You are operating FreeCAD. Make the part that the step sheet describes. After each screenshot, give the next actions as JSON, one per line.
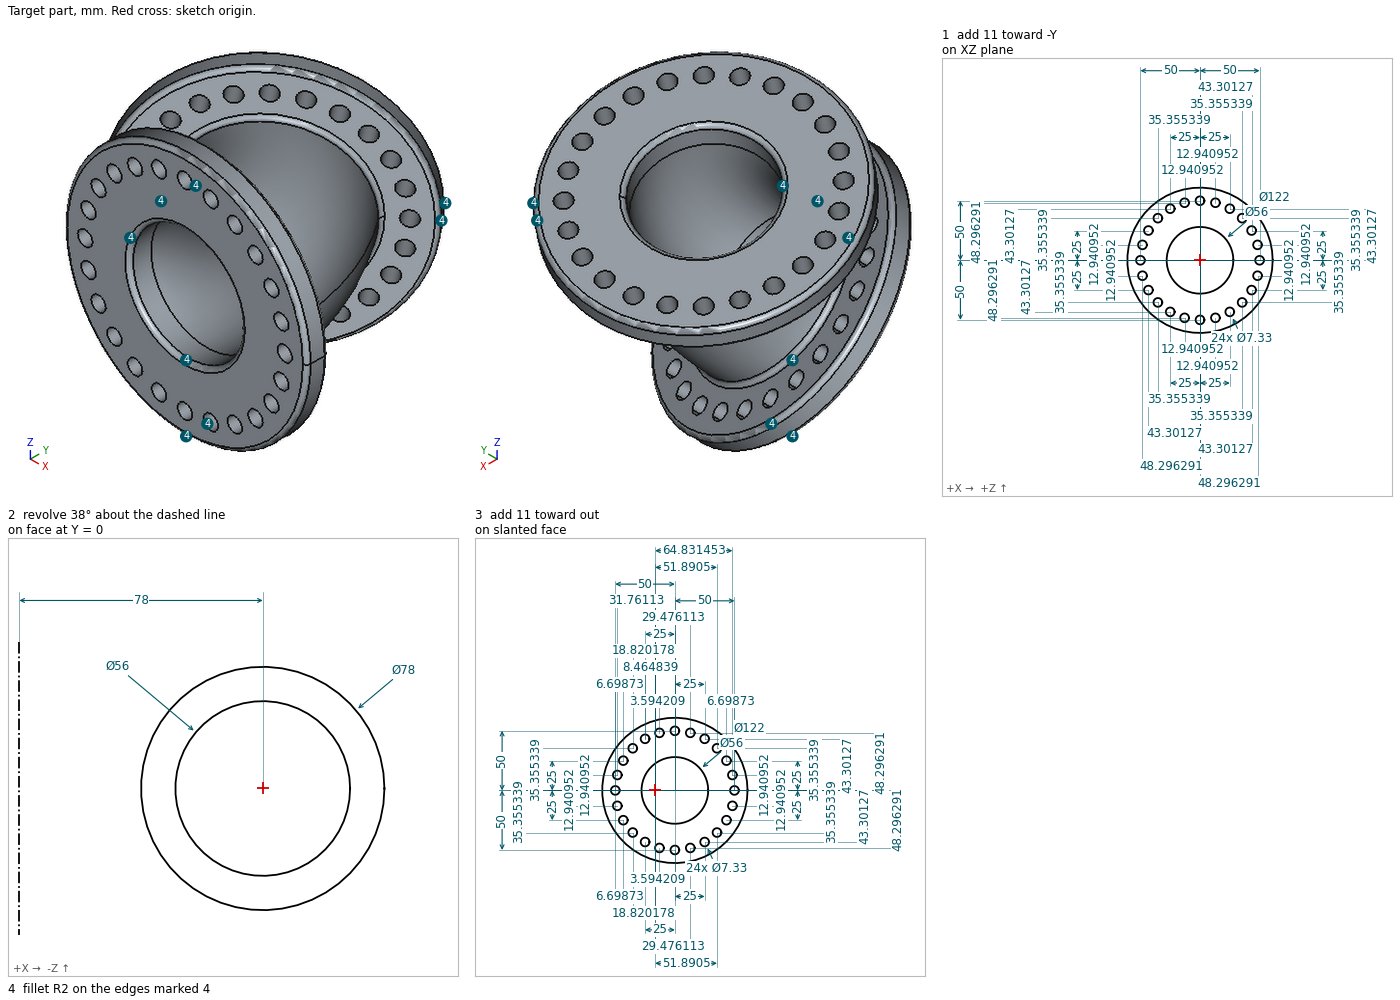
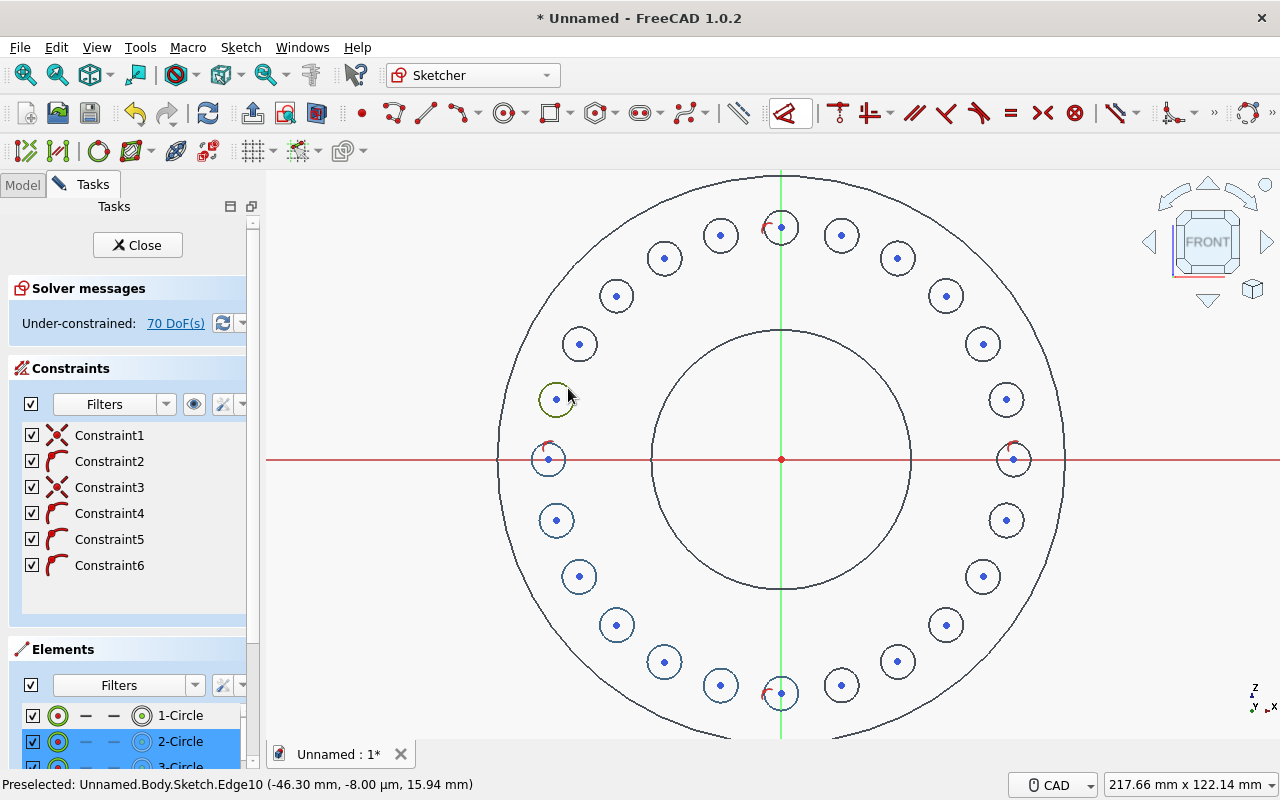
{"action": "left_click", "coordinate": [592, 332]}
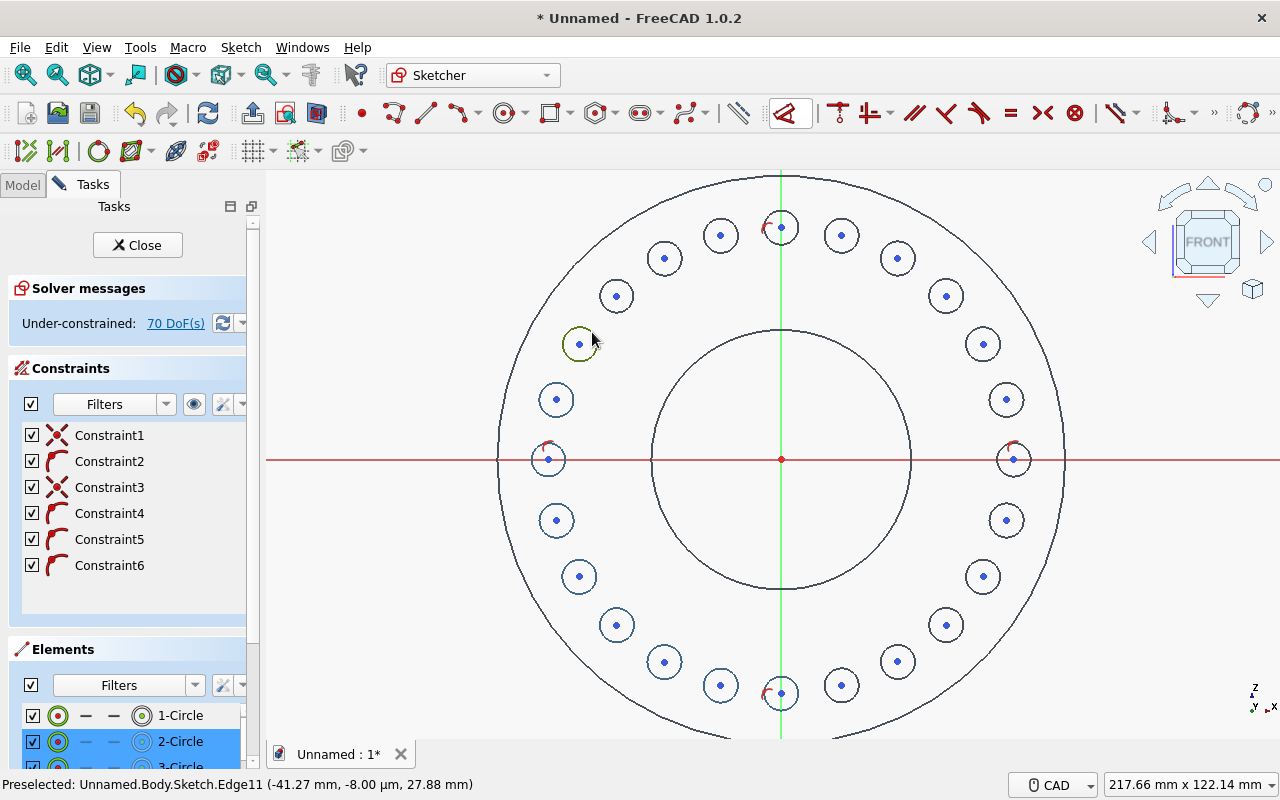
{"action": "left_click", "coordinate": [628, 284]}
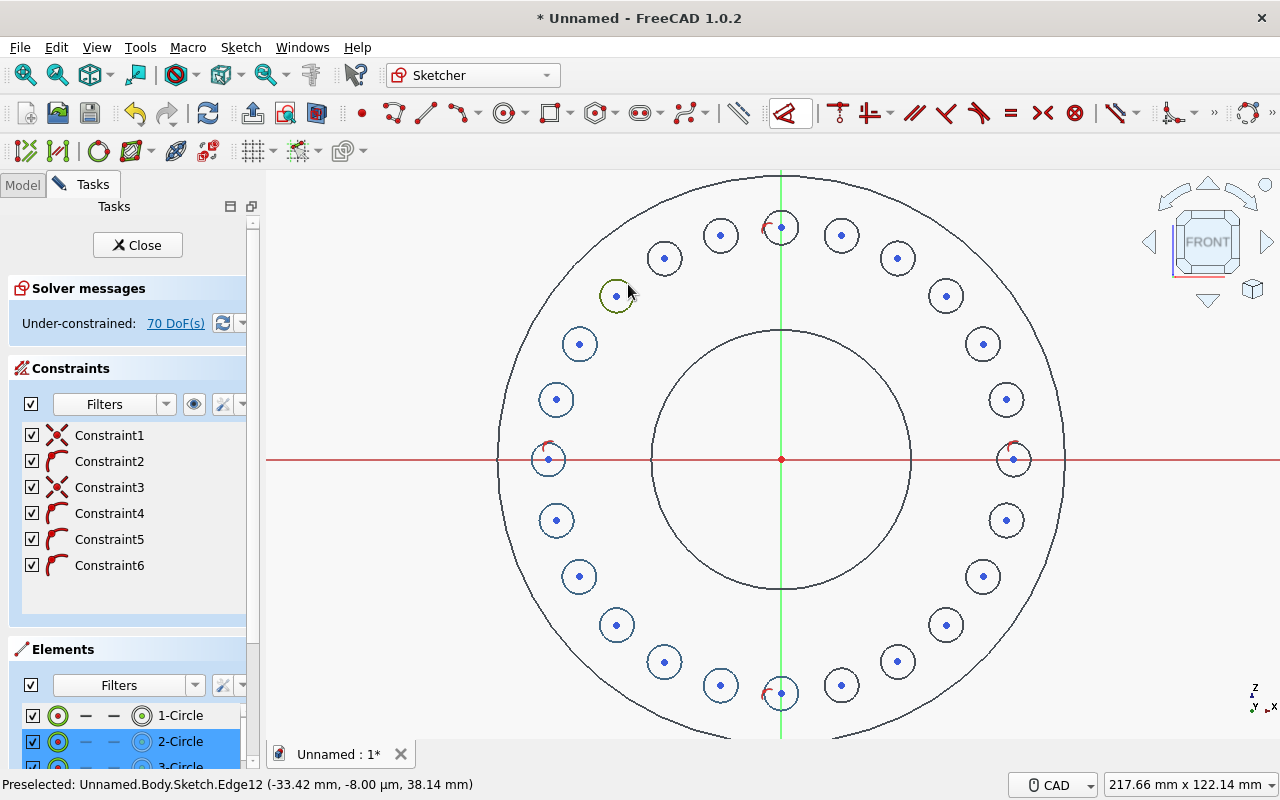
{"action": "left_click", "coordinate": [677, 246]}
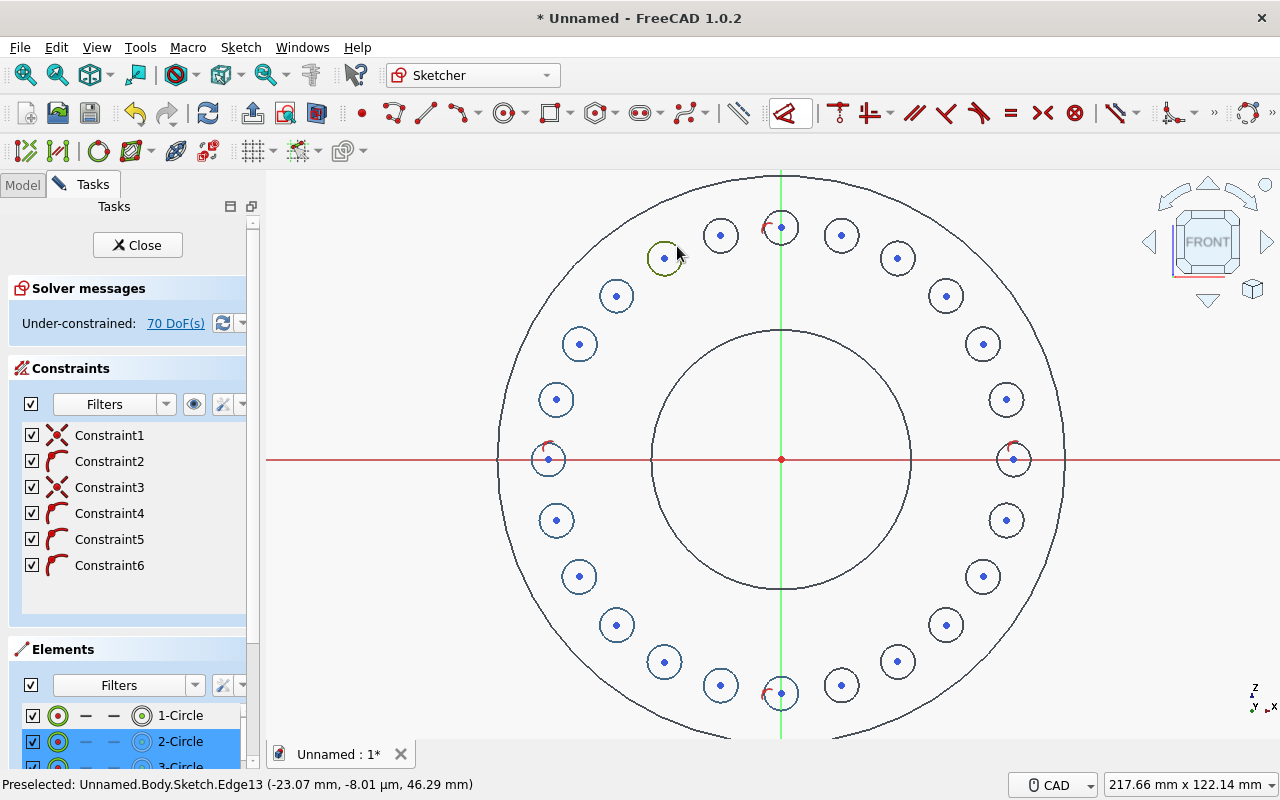
{"action": "left_click", "coordinate": [733, 224]}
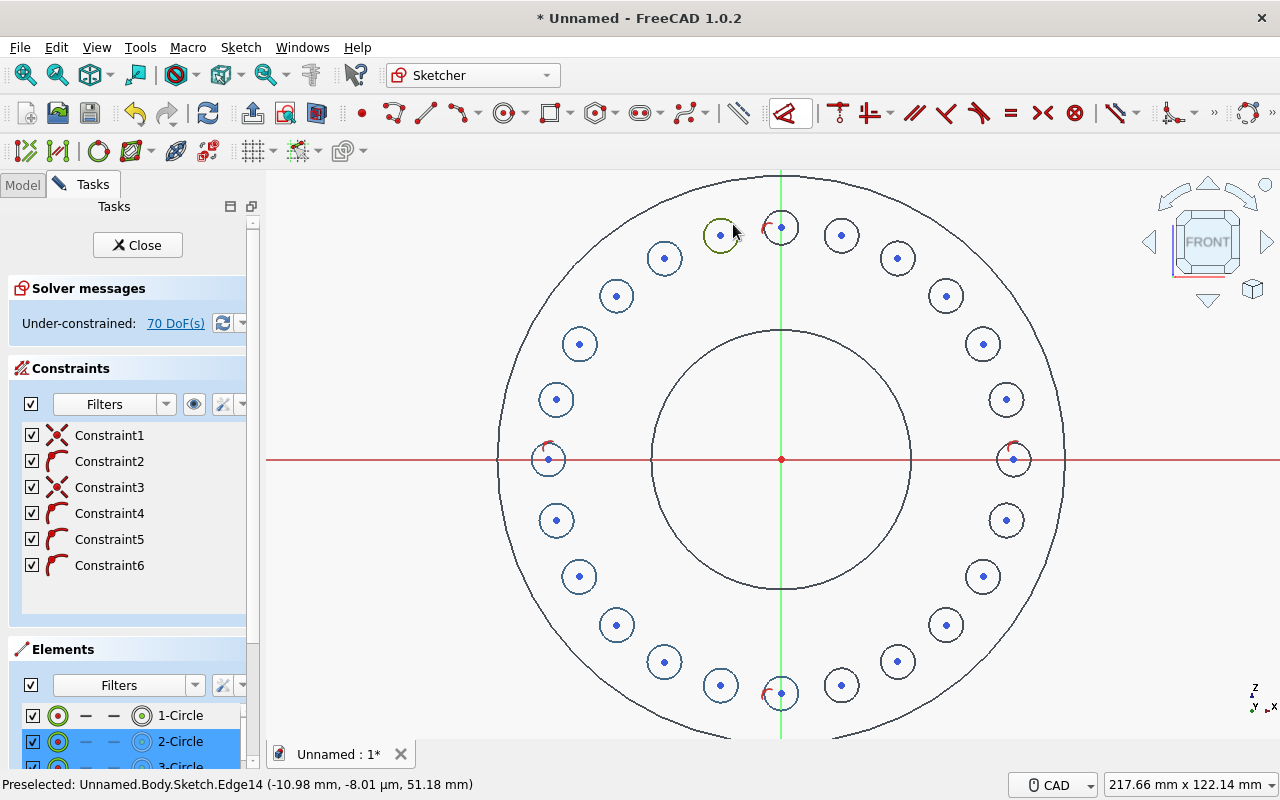
{"action": "left_click", "coordinate": [854, 673]}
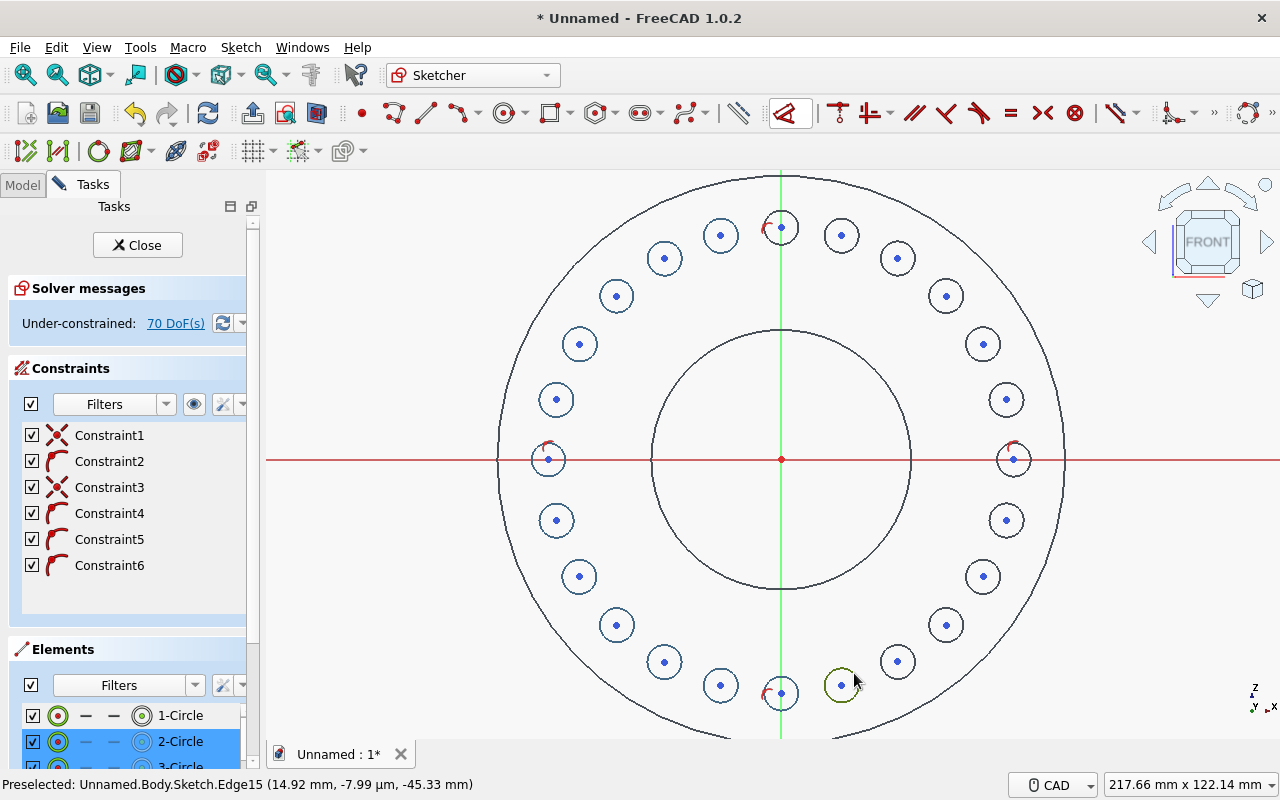
{"action": "left_click", "coordinate": [910, 650]}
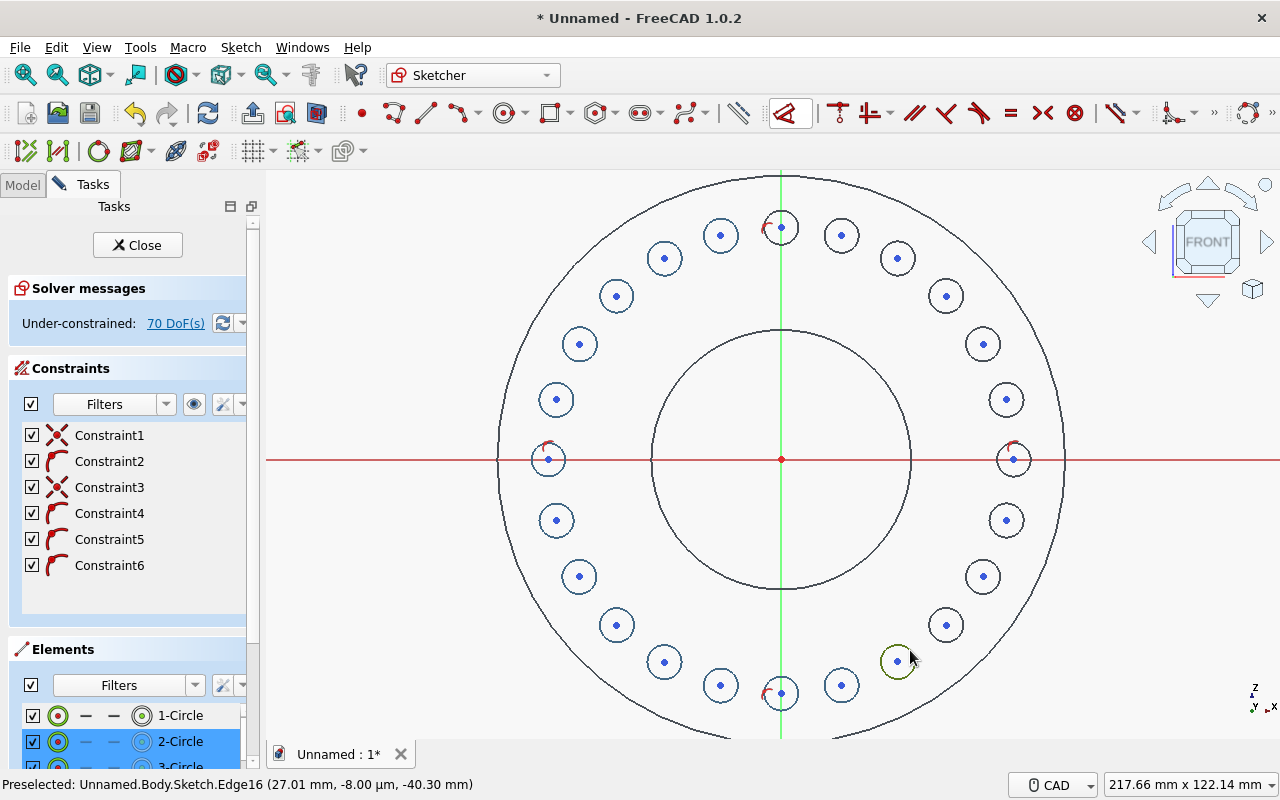
{"action": "left_click", "coordinate": [958, 613]}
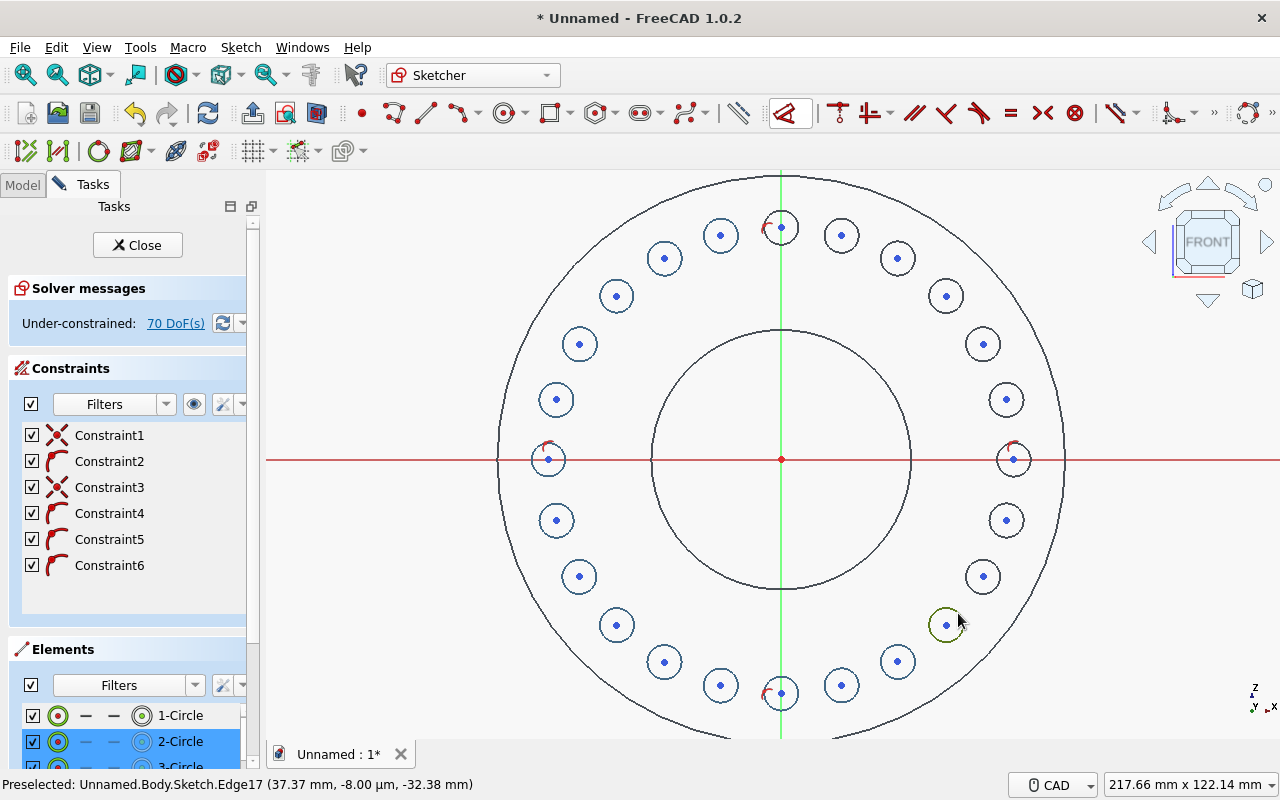
{"action": "left_click", "coordinate": [995, 565]}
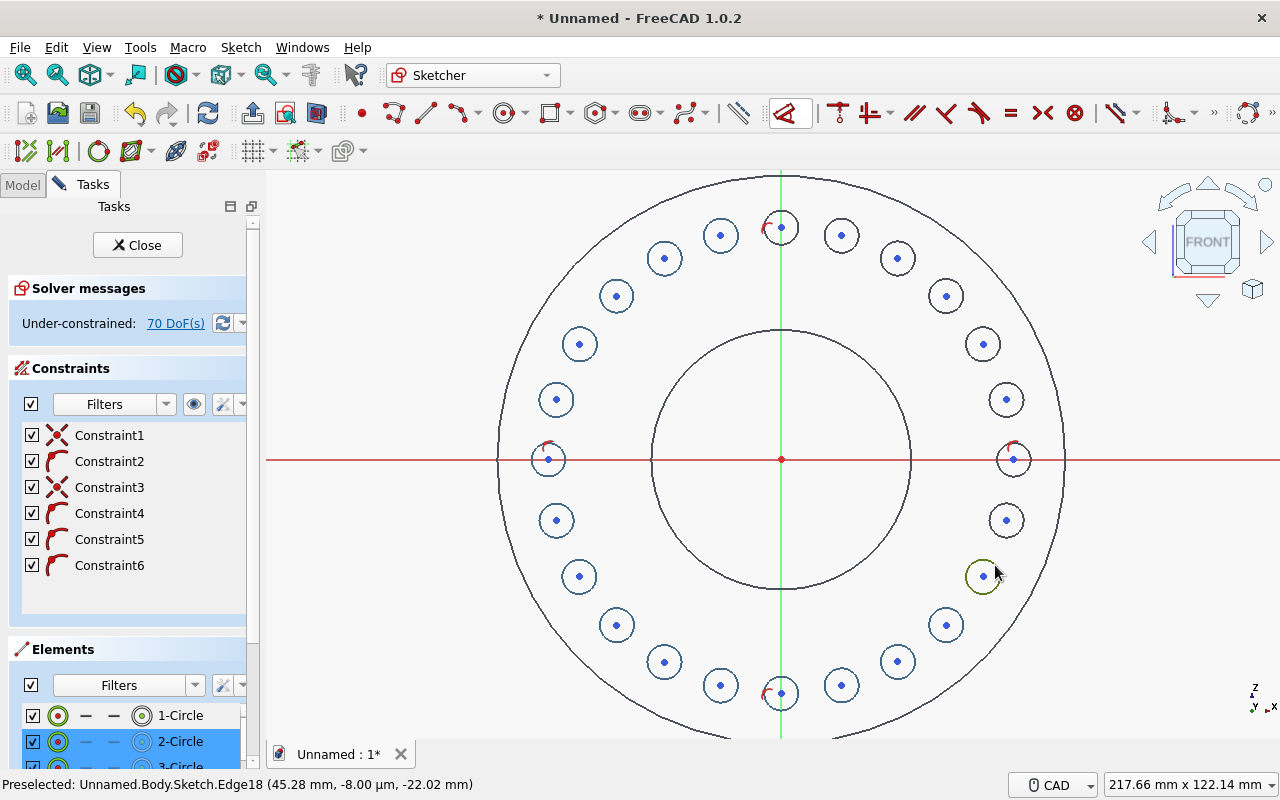
{"action": "left_click", "coordinate": [1019, 508]}